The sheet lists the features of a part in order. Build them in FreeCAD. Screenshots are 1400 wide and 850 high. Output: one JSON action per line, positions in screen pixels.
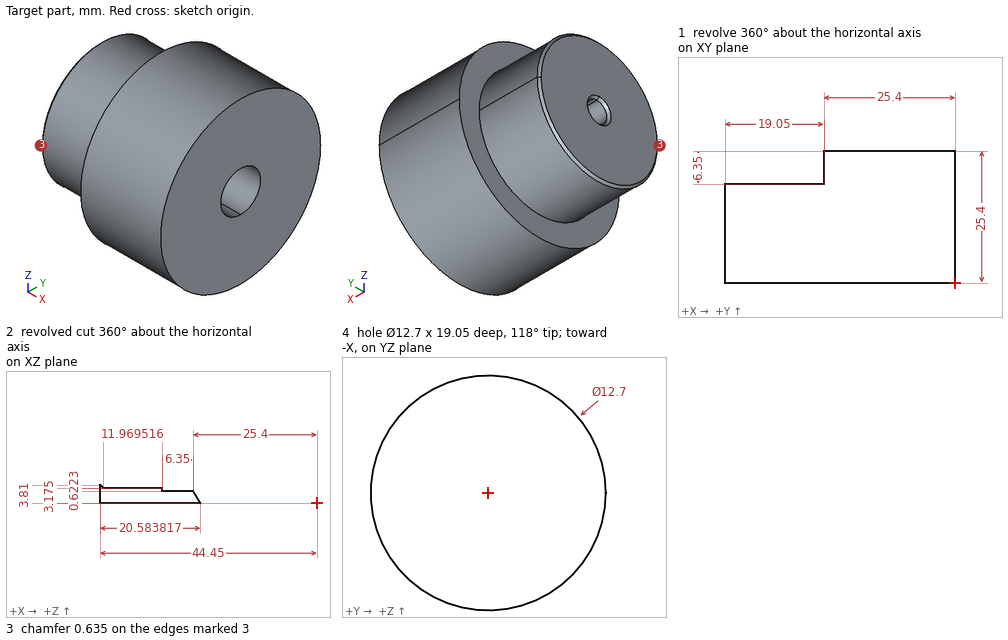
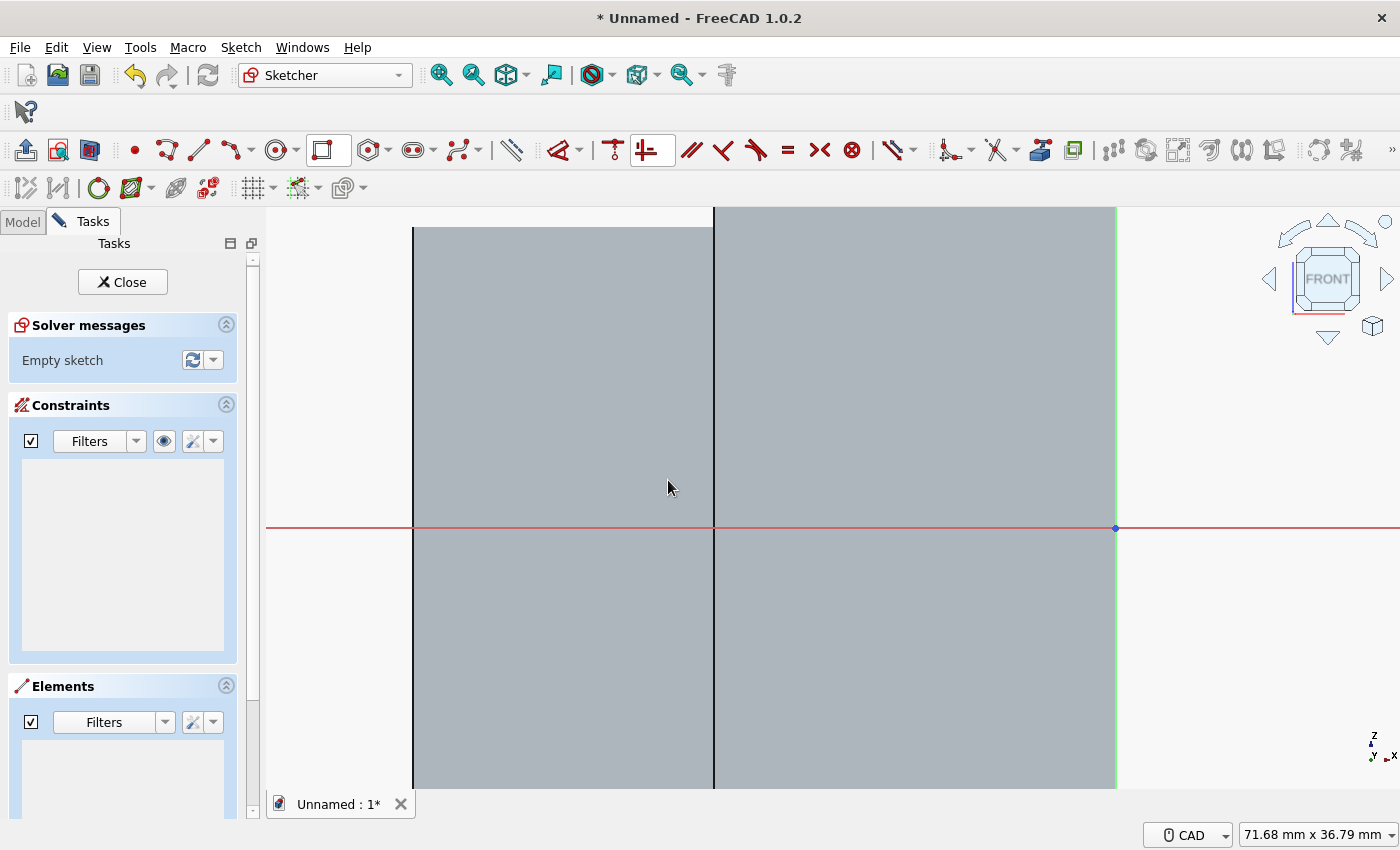
{"action": "left_click", "coordinate": [168, 150]}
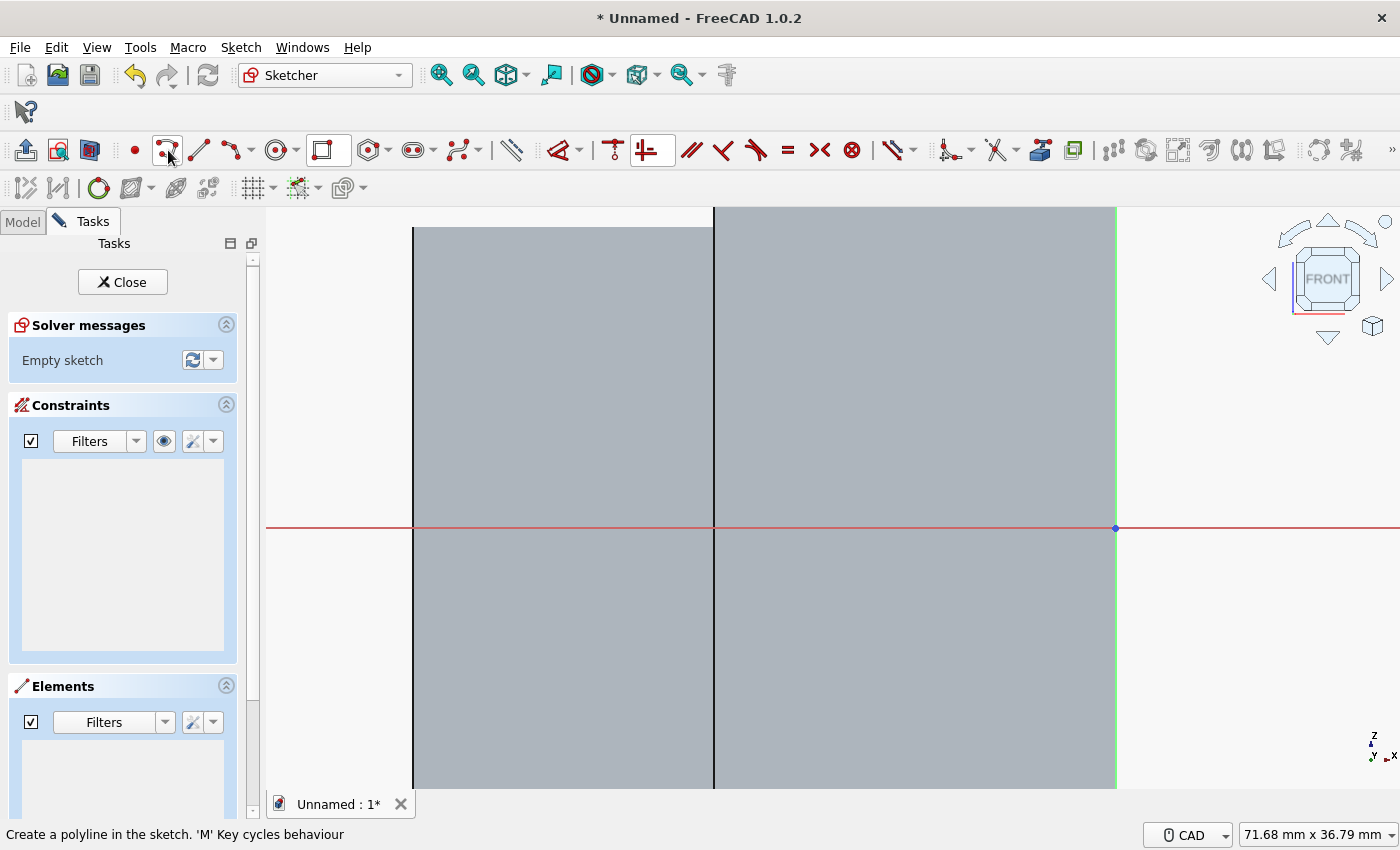
{"action": "left_click", "coordinate": [738, 528]}
{"action": "left_click", "coordinate": [413, 519]}
{"action": "left_click", "coordinate": [413, 468]}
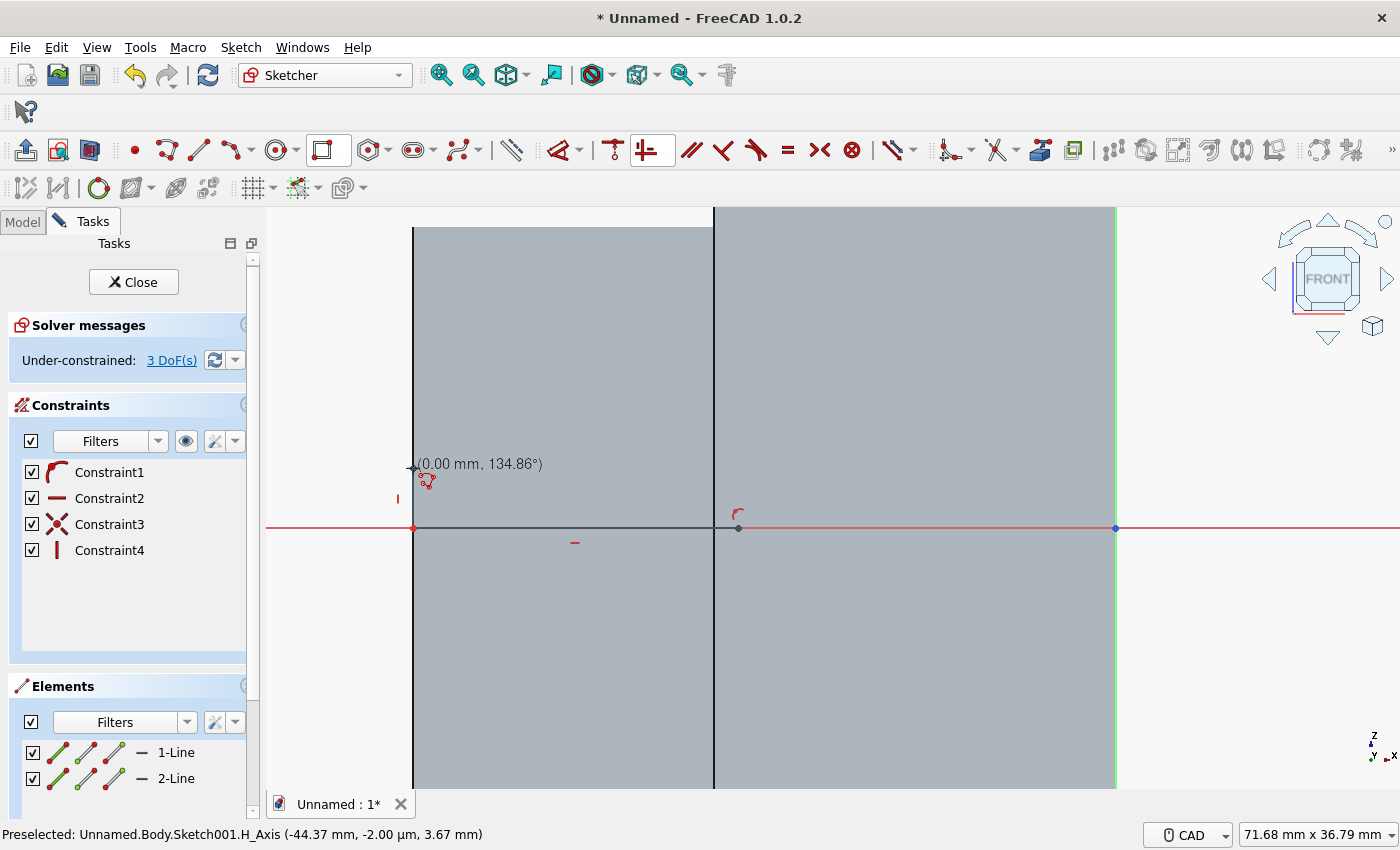
{"action": "scroll", "coordinate": [424, 478], "scroll_direction": "up", "scroll_amount": 2}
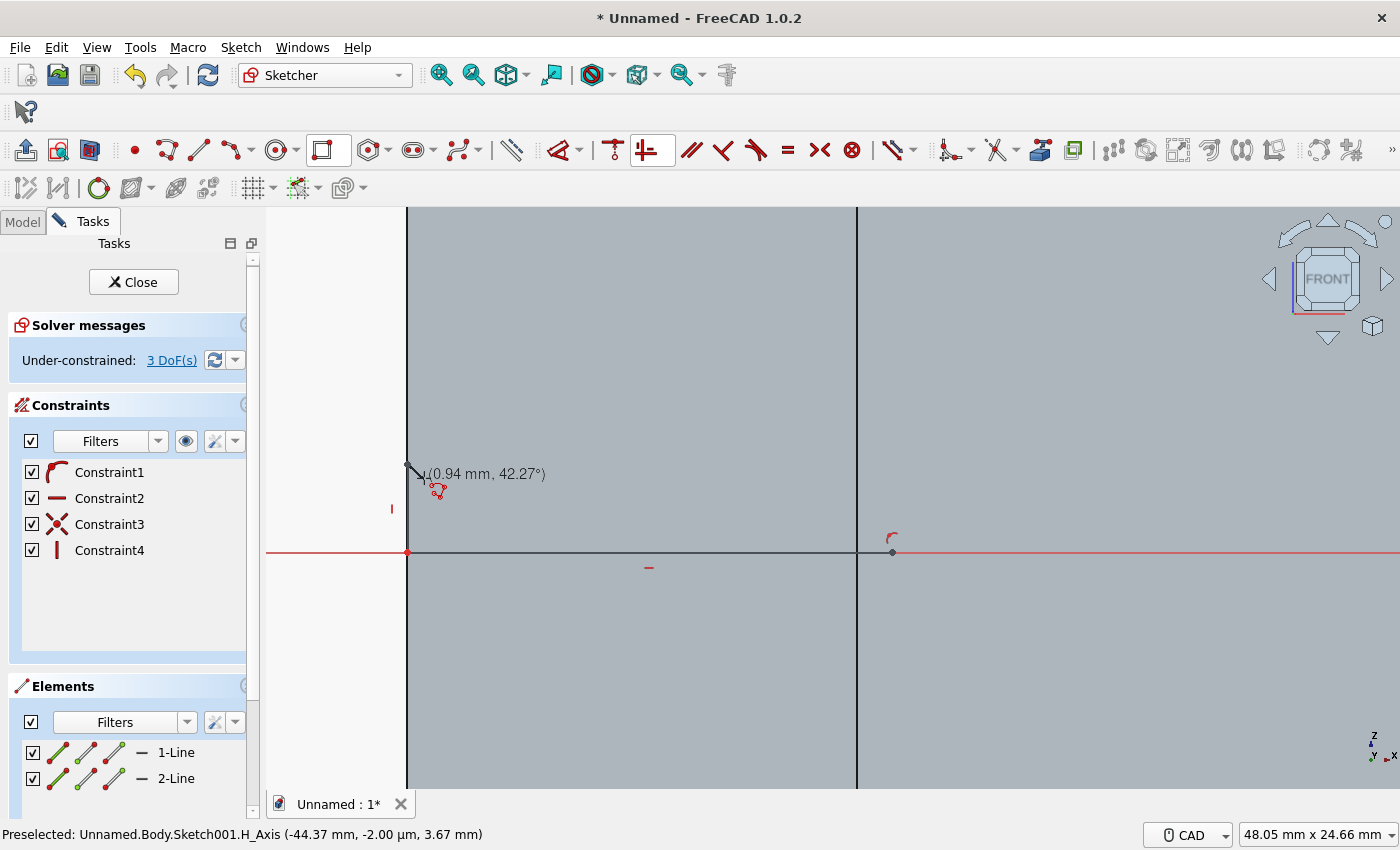
{"action": "left_click", "coordinate": [424, 478]}
{"action": "left_click", "coordinate": [707, 478]}
{"action": "left_click", "coordinate": [707, 492]}
{"action": "left_click", "coordinate": [857, 492]}
{"action": "left_click", "coordinate": [892, 553]}
{"action": "key", "text": "Escape"}
{"action": "key", "text": "Escape"}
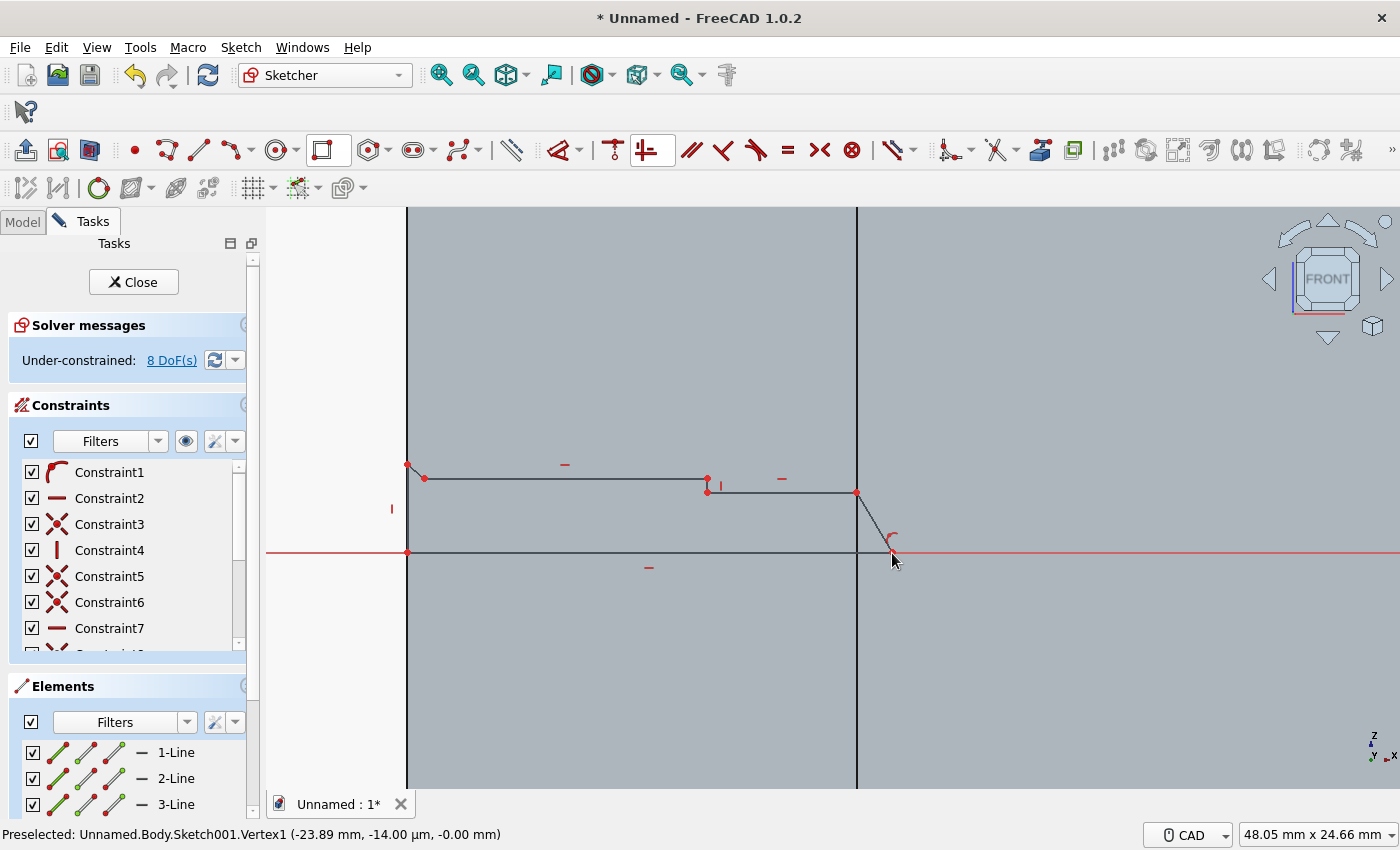
{"action": "left_click", "coordinate": [558, 150]}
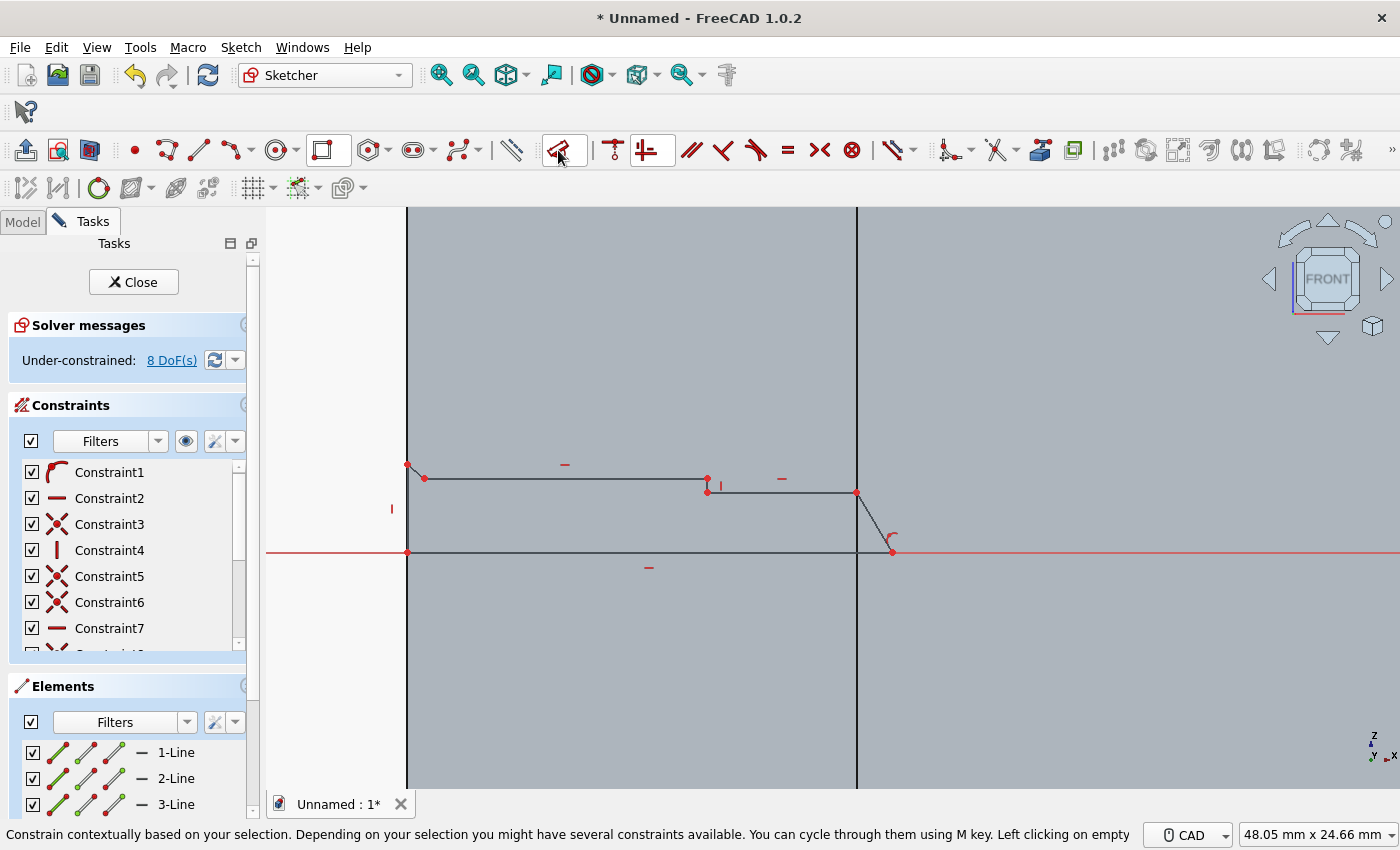
{"action": "left_click", "coordinate": [408, 526]}
{"action": "left_click", "coordinate": [374, 508]}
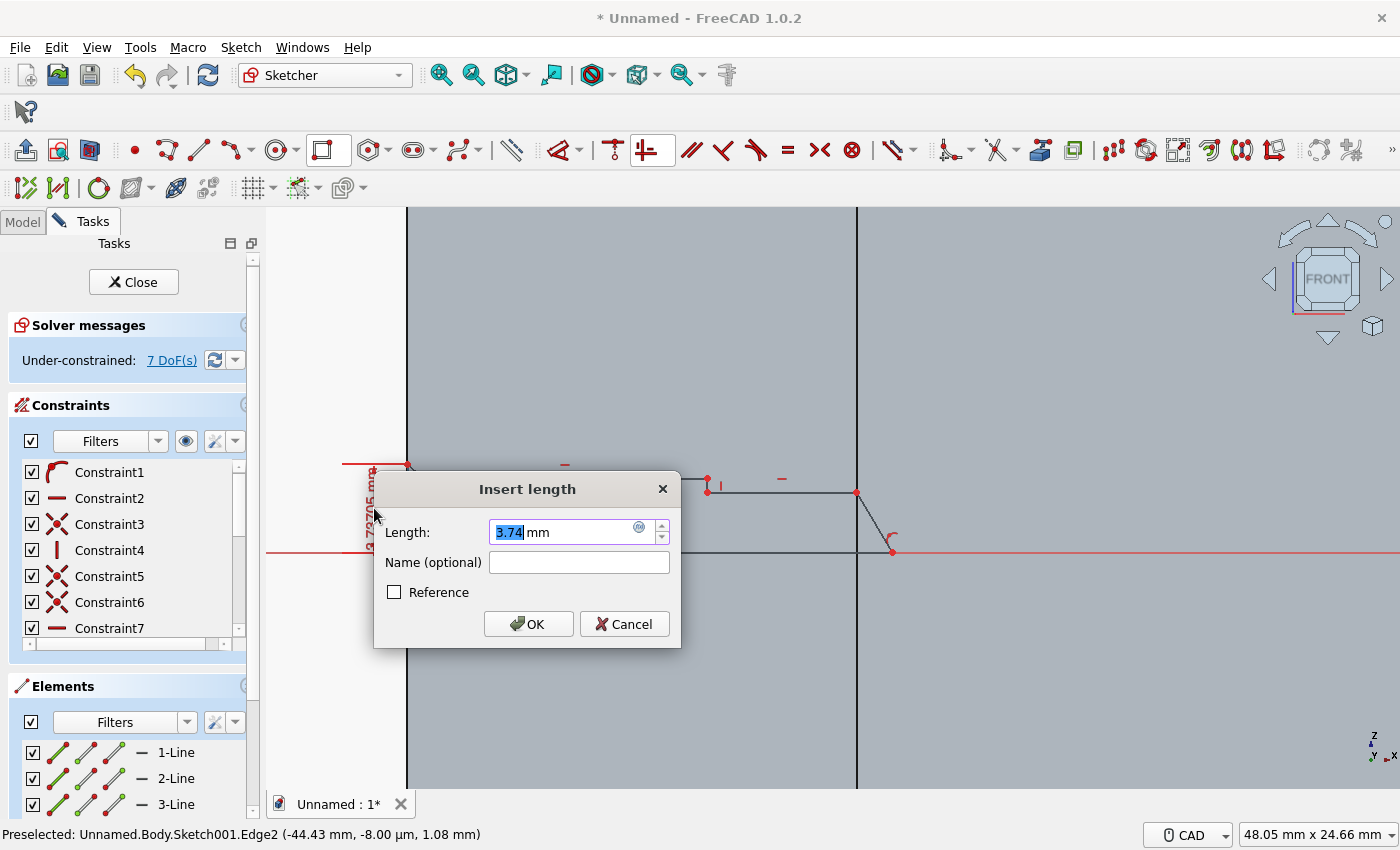
{"action": "type", "text": "3.81"}
{"action": "key", "text": "Return"}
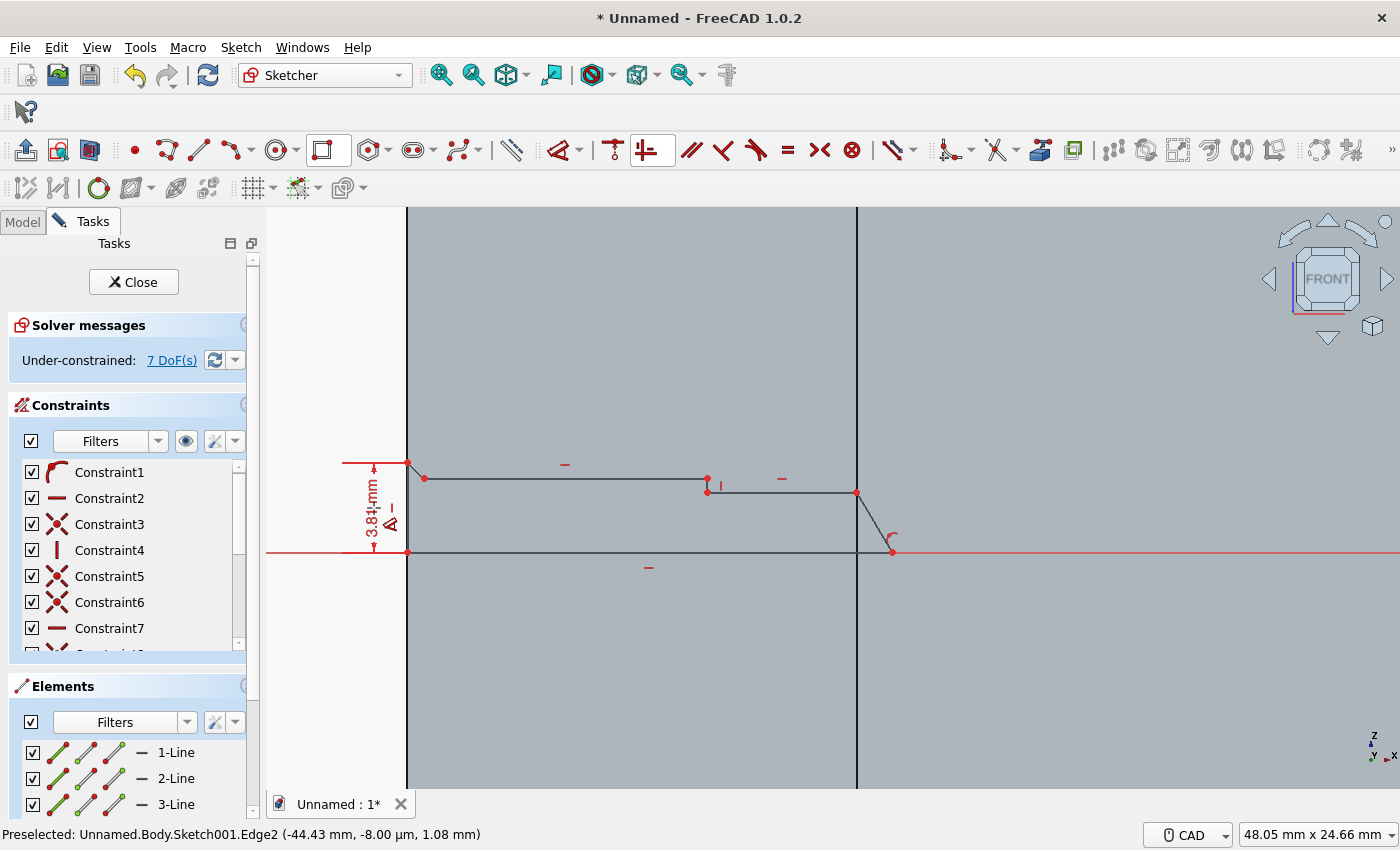
{"action": "left_click", "coordinate": [752, 493]}
{"action": "left_click", "coordinate": [782, 459]}